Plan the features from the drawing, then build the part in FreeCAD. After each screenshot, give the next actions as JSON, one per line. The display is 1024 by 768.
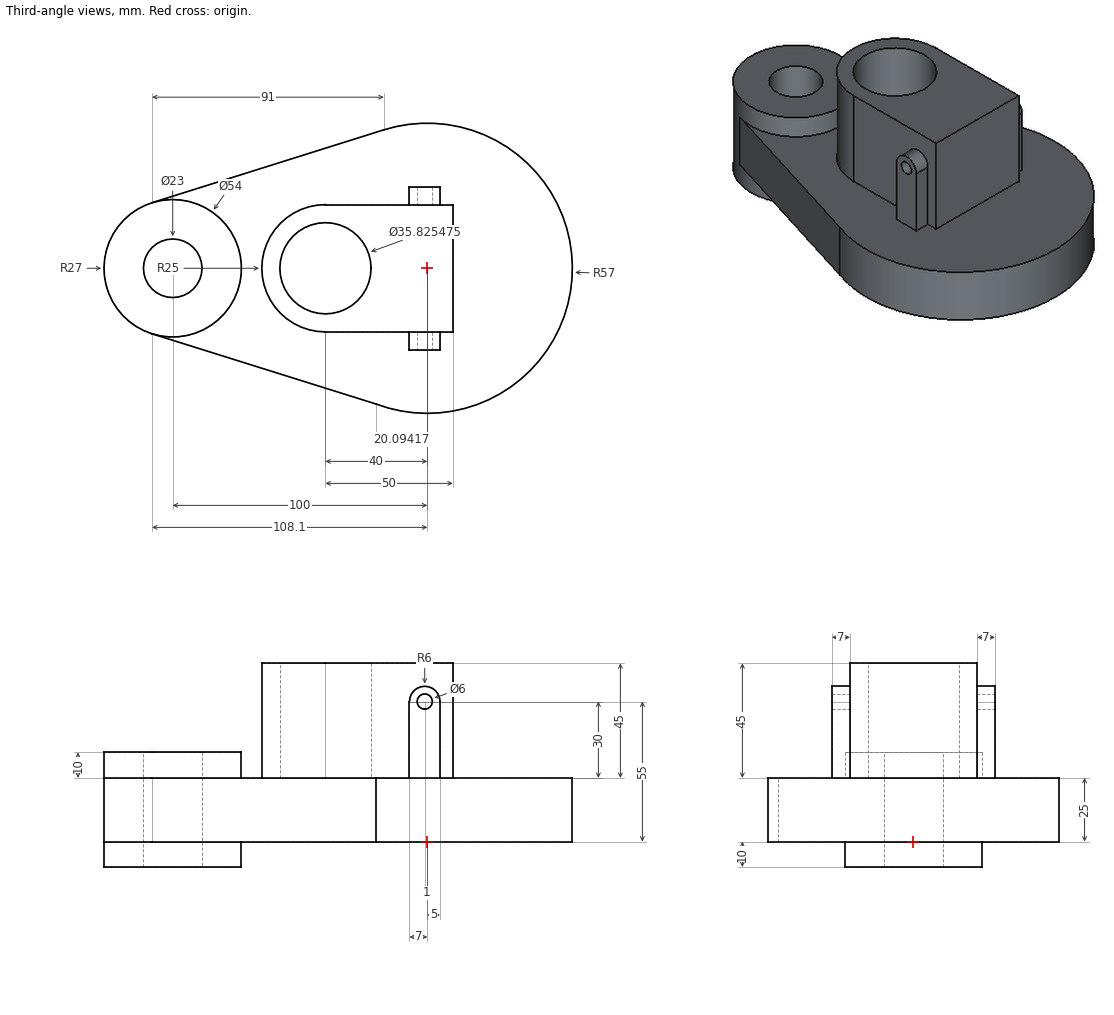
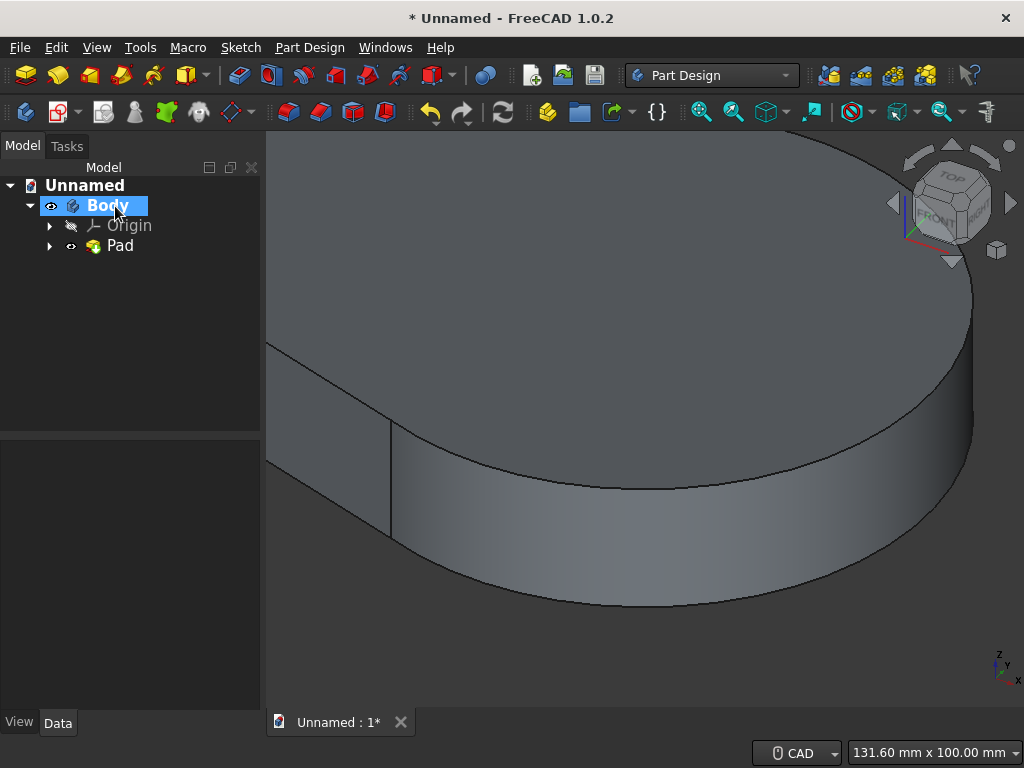
{"action": "key", "text": "v f"}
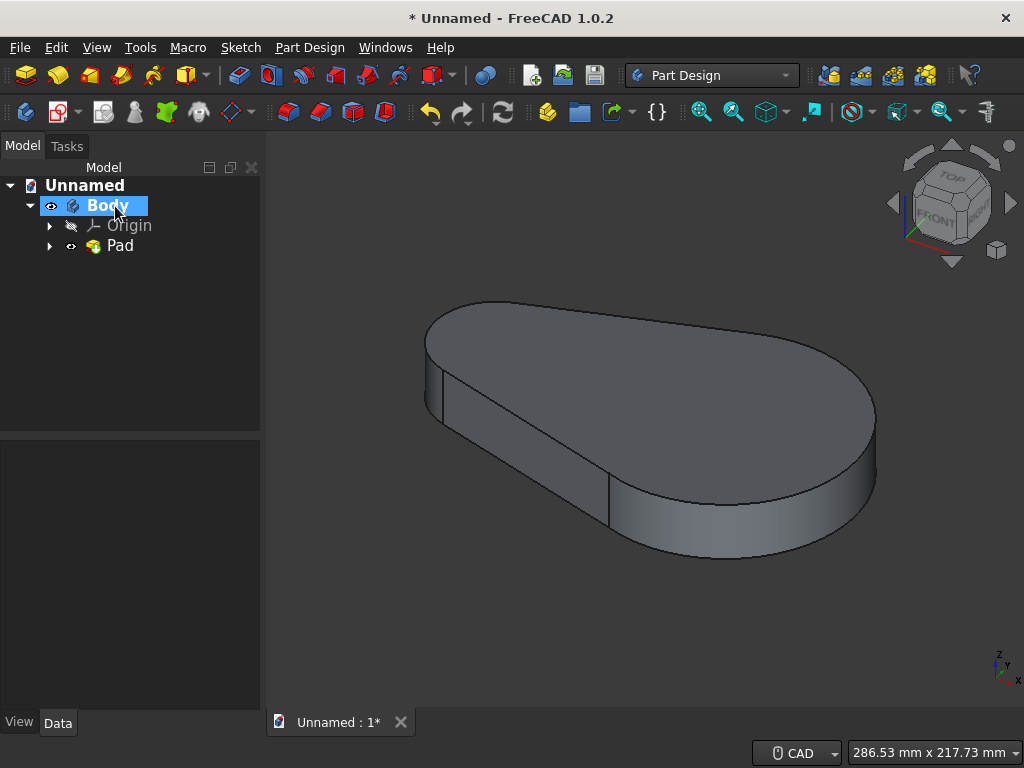
{"action": "left_click", "coordinate": [705, 411]}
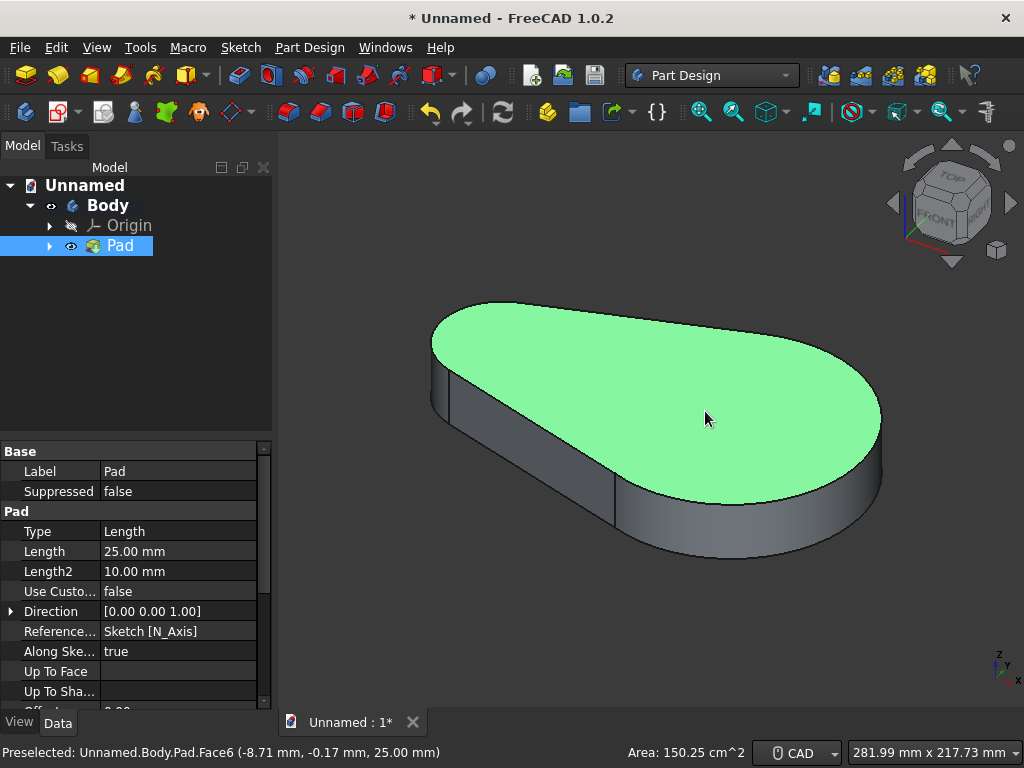
{"action": "left_click", "coordinate": [58, 112]}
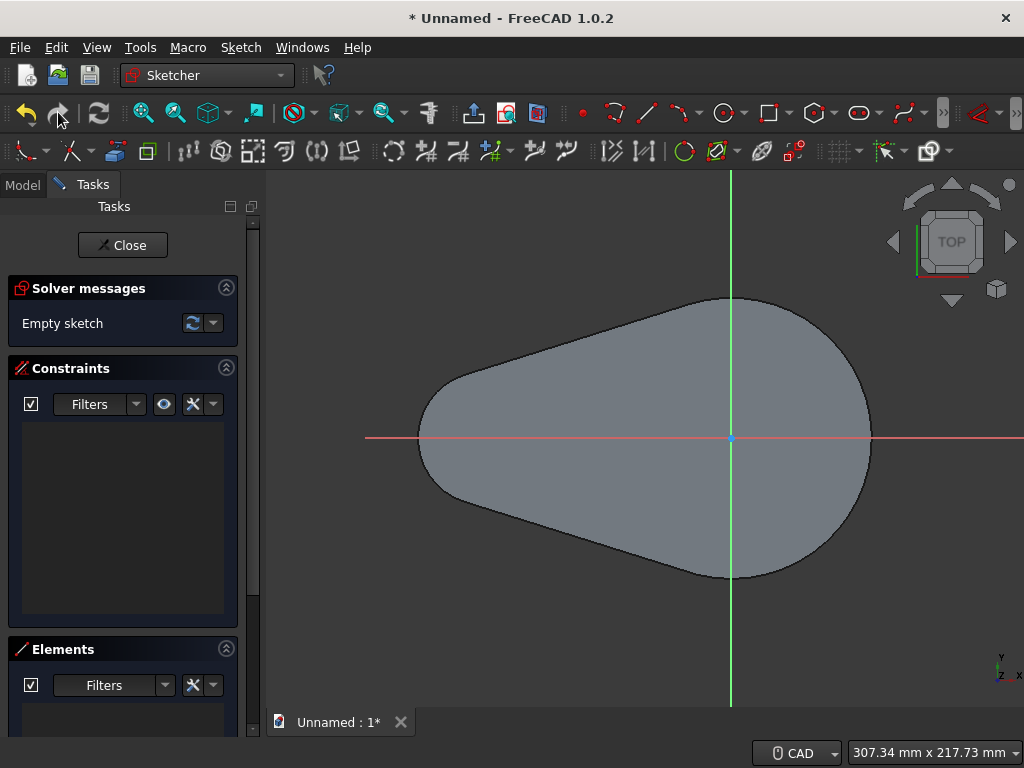
{"action": "key", "text": "g c"}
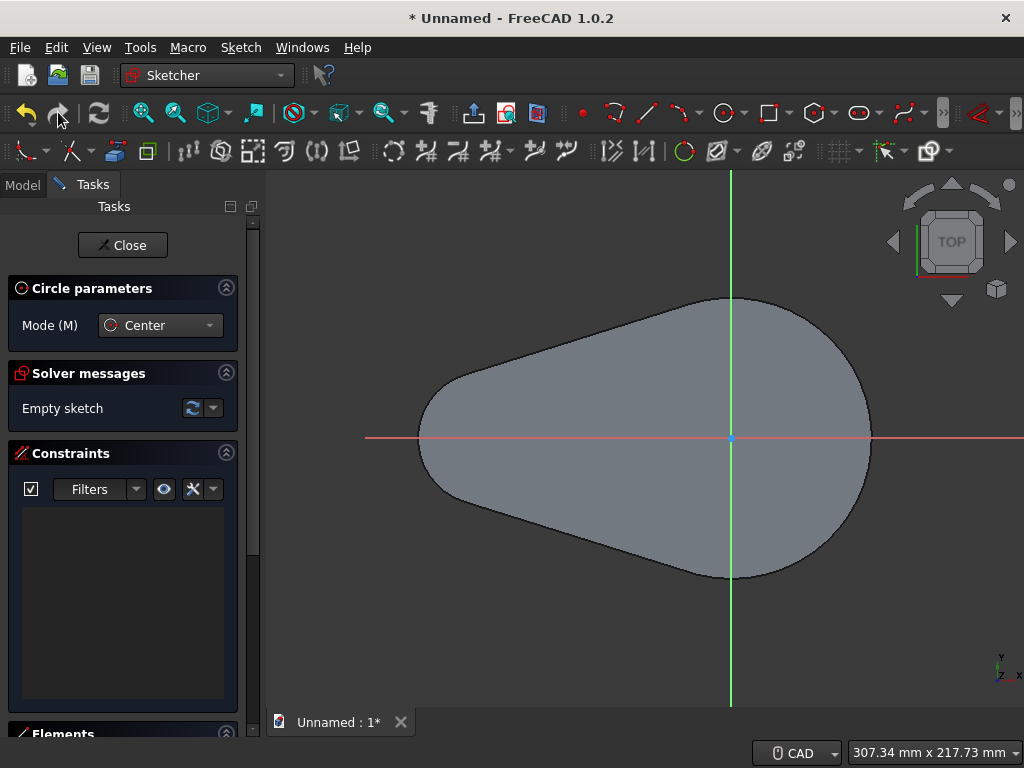
{"action": "left_click", "coordinate": [485, 438]}
{"action": "left_click", "coordinate": [532, 391]}
{"action": "key", "text": "Escape"}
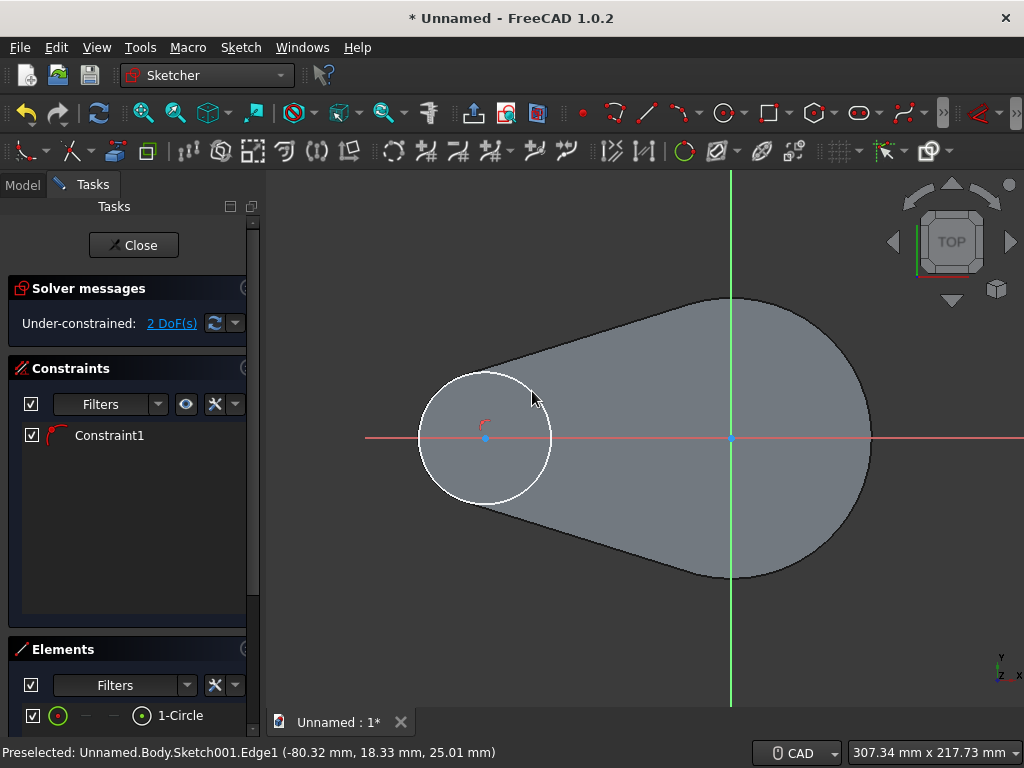
{"action": "key", "text": "d"}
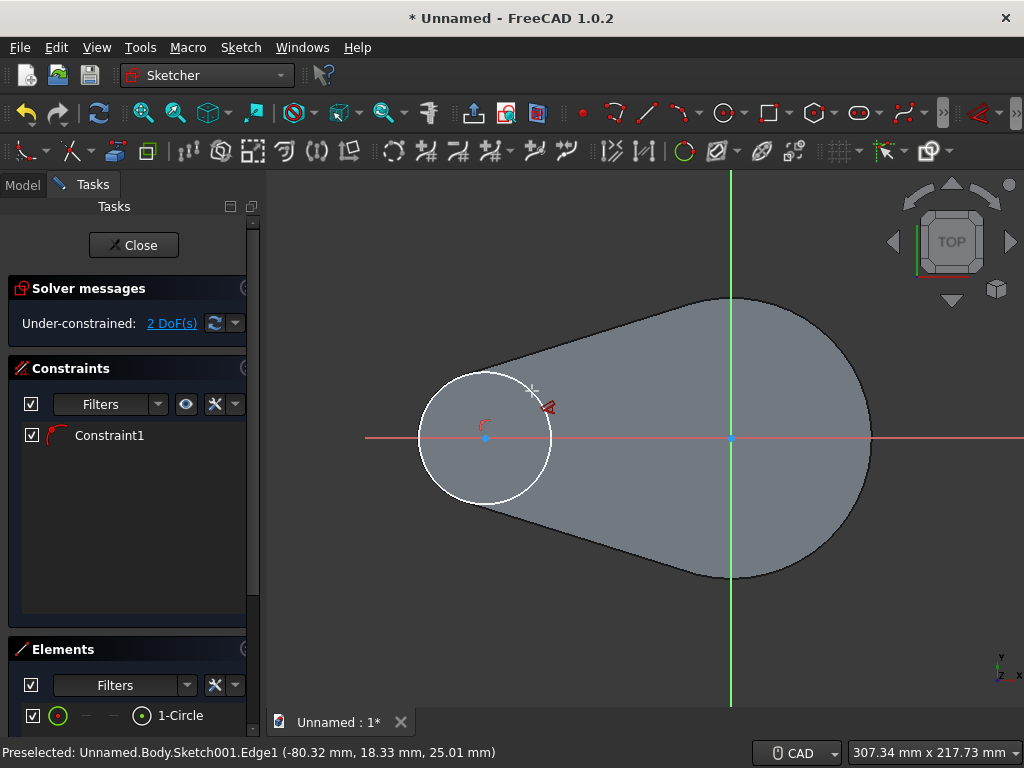
{"action": "left_click", "coordinate": [532, 392]}
{"action": "left_click", "coordinate": [555, 370]}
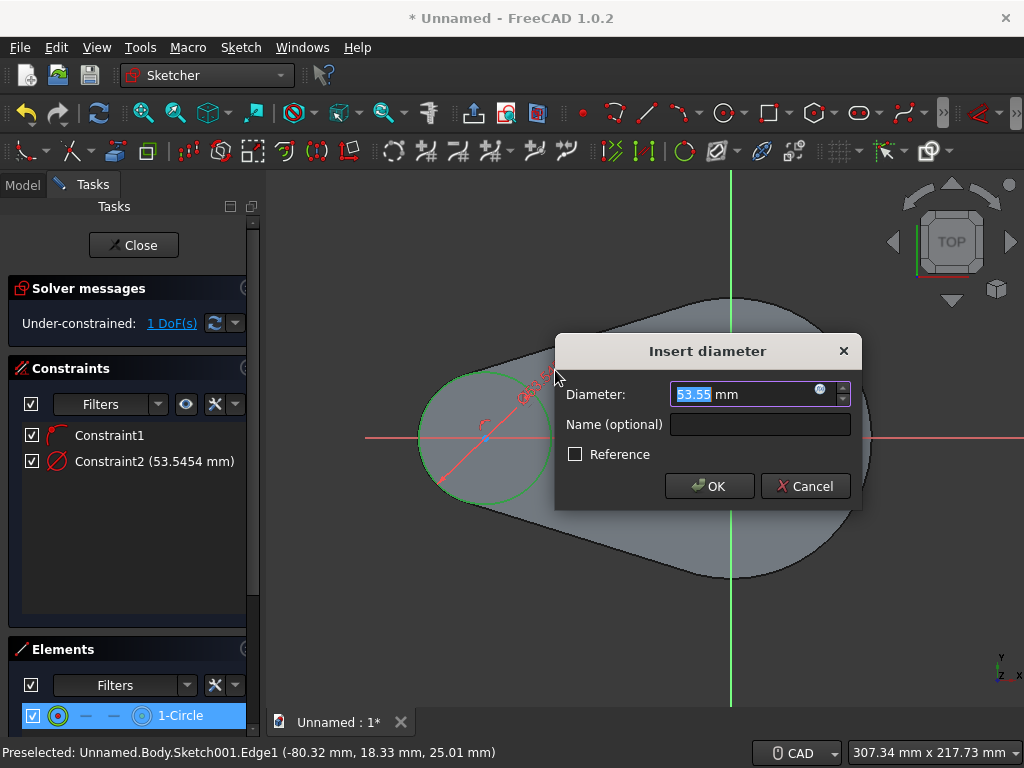
{"action": "type", "text": "54"}
{"action": "key", "text": "Return"}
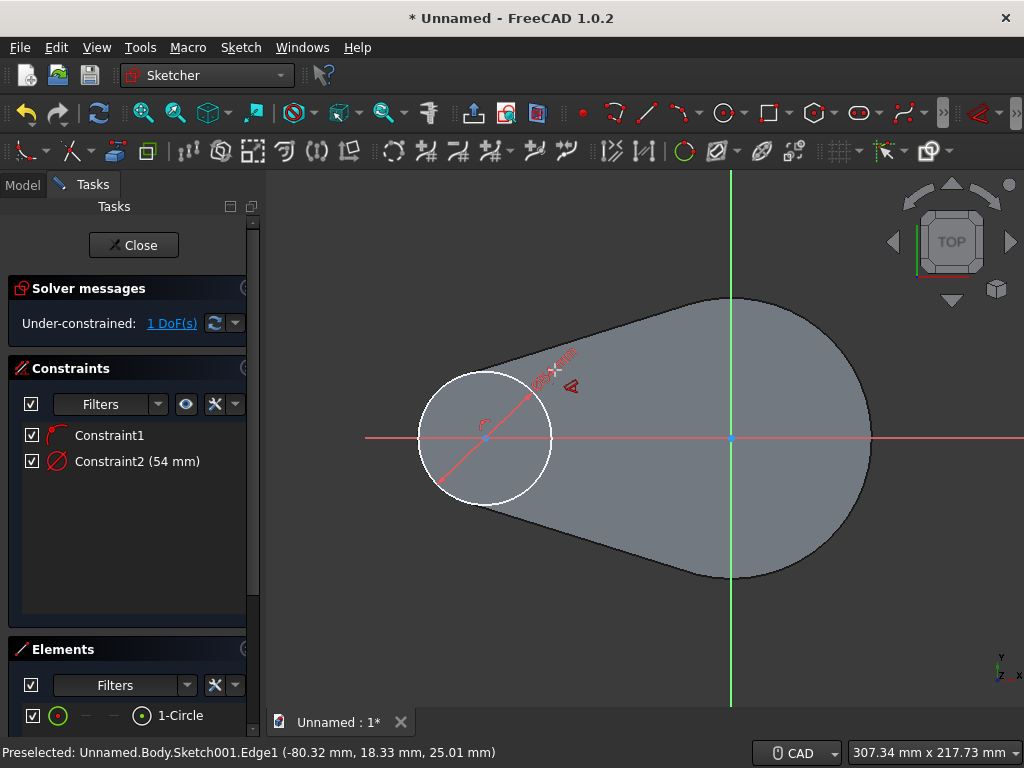
{"action": "left_click", "coordinate": [485, 438]}
{"action": "left_click", "coordinate": [608, 472]}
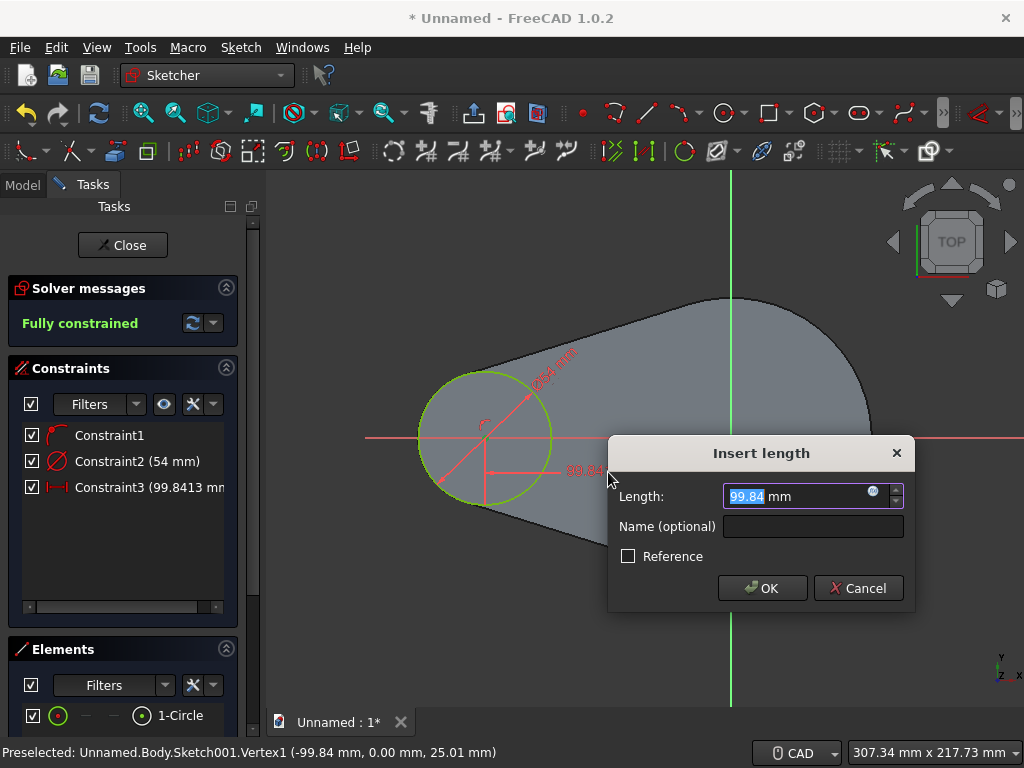
{"action": "type", "text": "100"}
{"action": "key", "text": "Return"}
{"action": "key", "text": "Escape"}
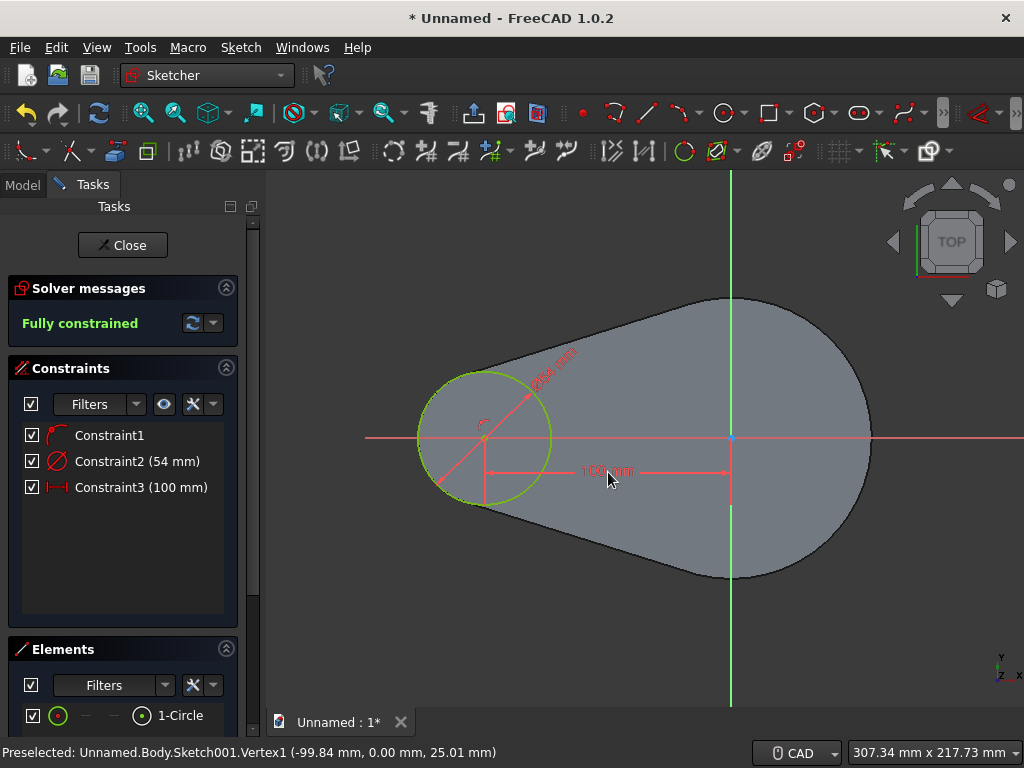
{"action": "left_click", "coordinate": [123, 245]}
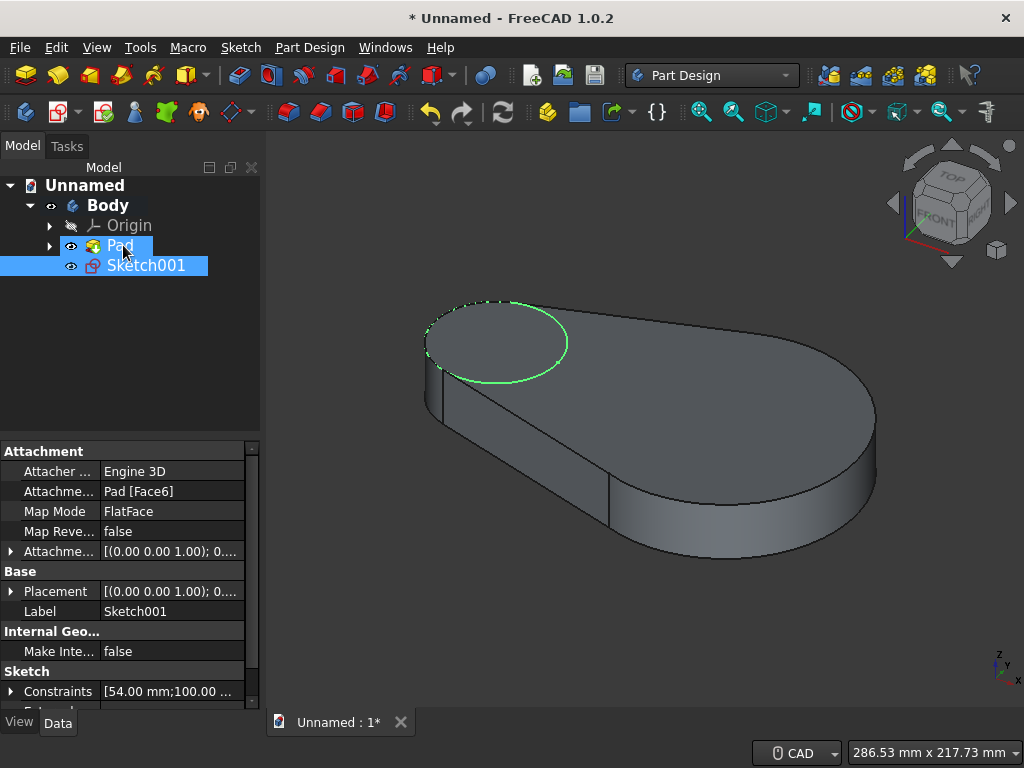
{"action": "left_click", "coordinate": [26, 76]}